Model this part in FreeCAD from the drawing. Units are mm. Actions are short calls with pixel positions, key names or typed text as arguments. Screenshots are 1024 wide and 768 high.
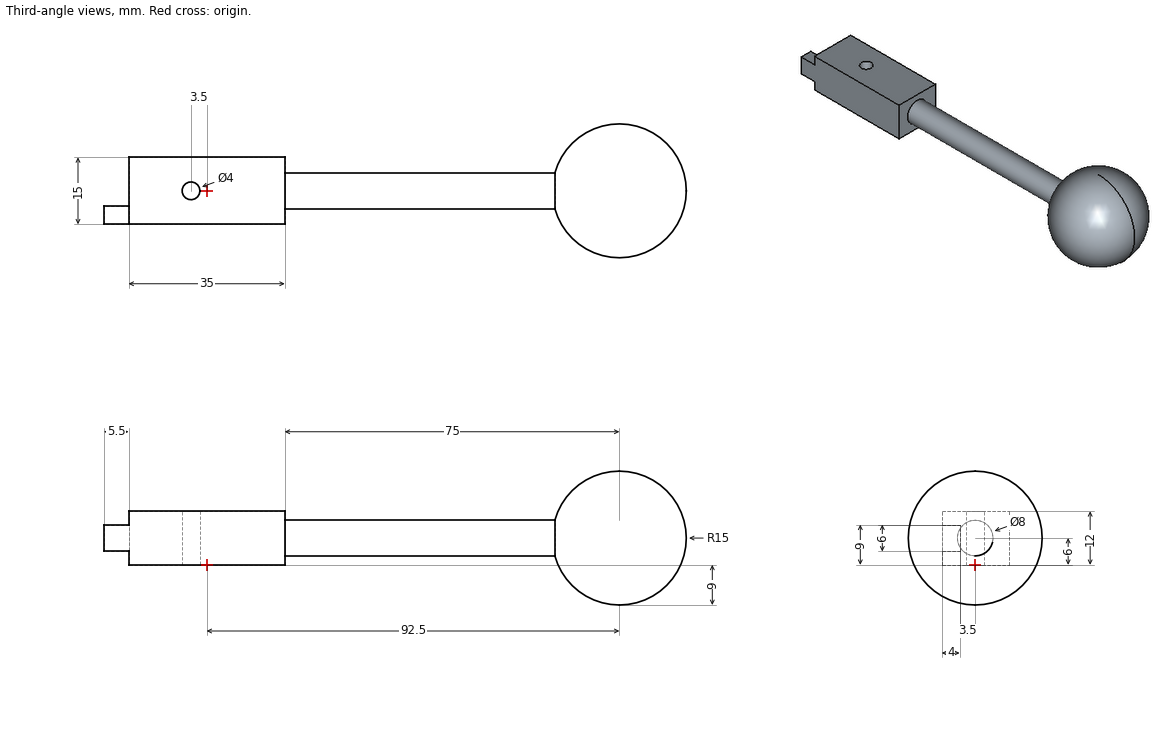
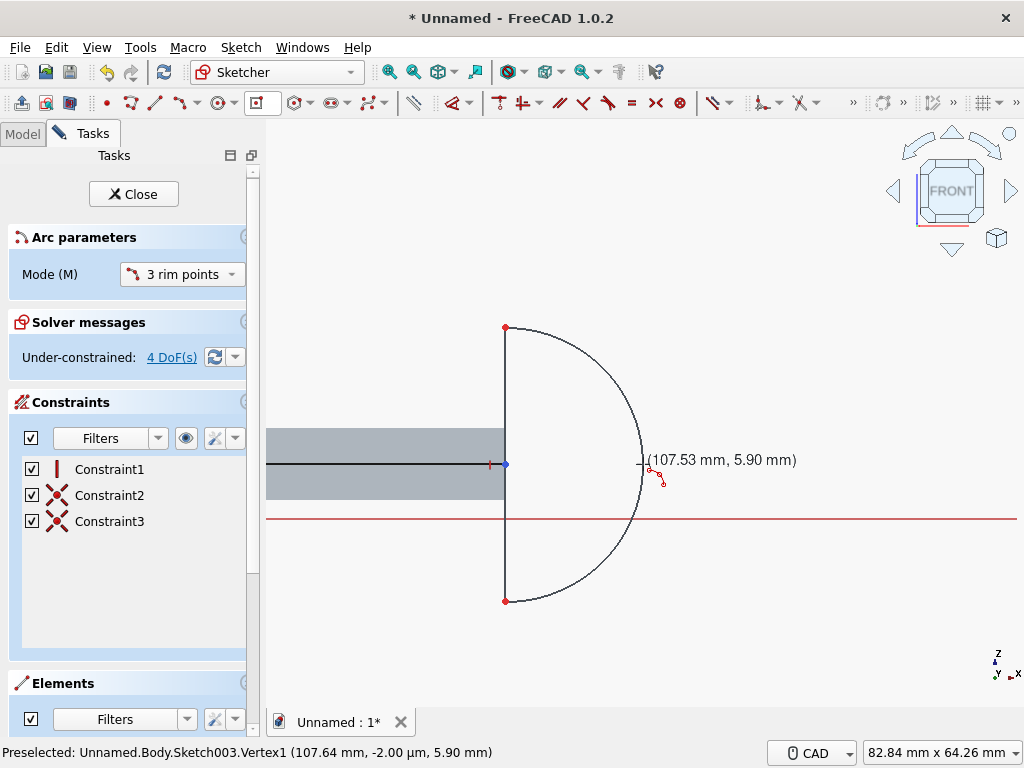
click(156, 104)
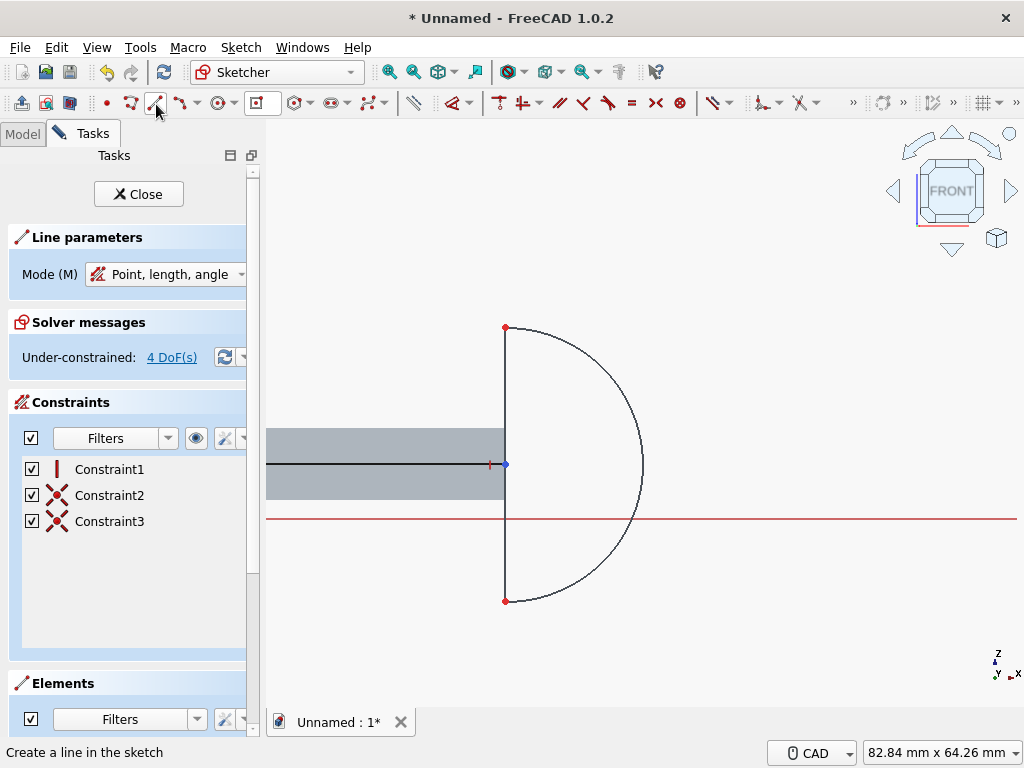
click(505, 299)
click(505, 217)
key(Escape)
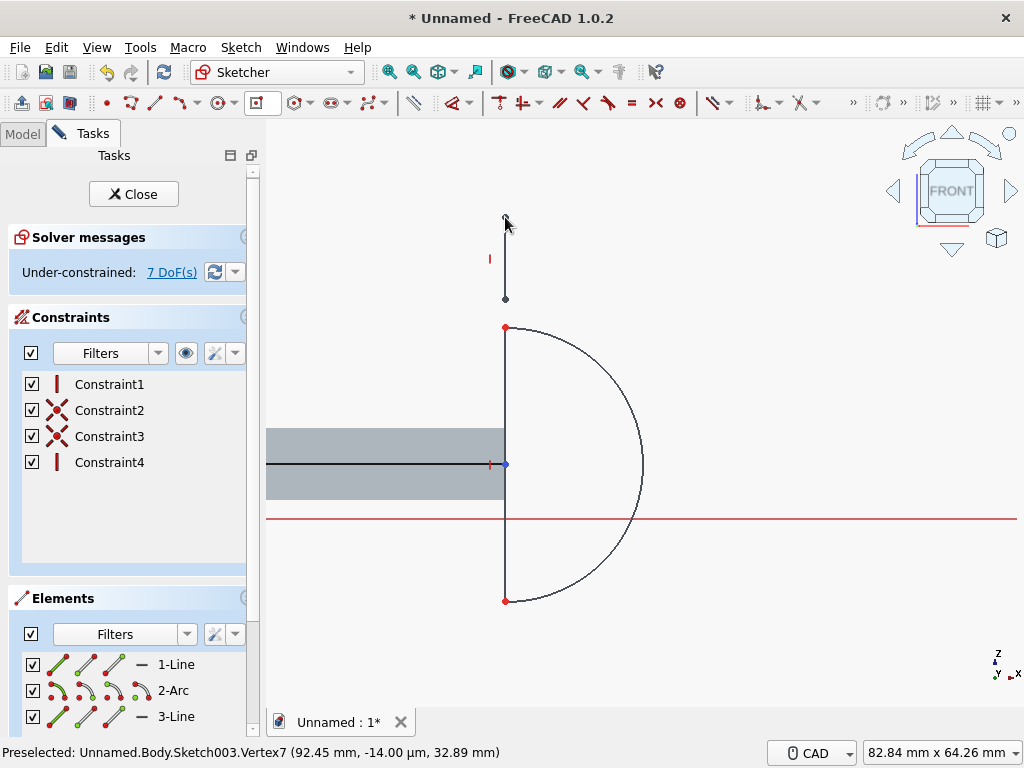
click(505, 275)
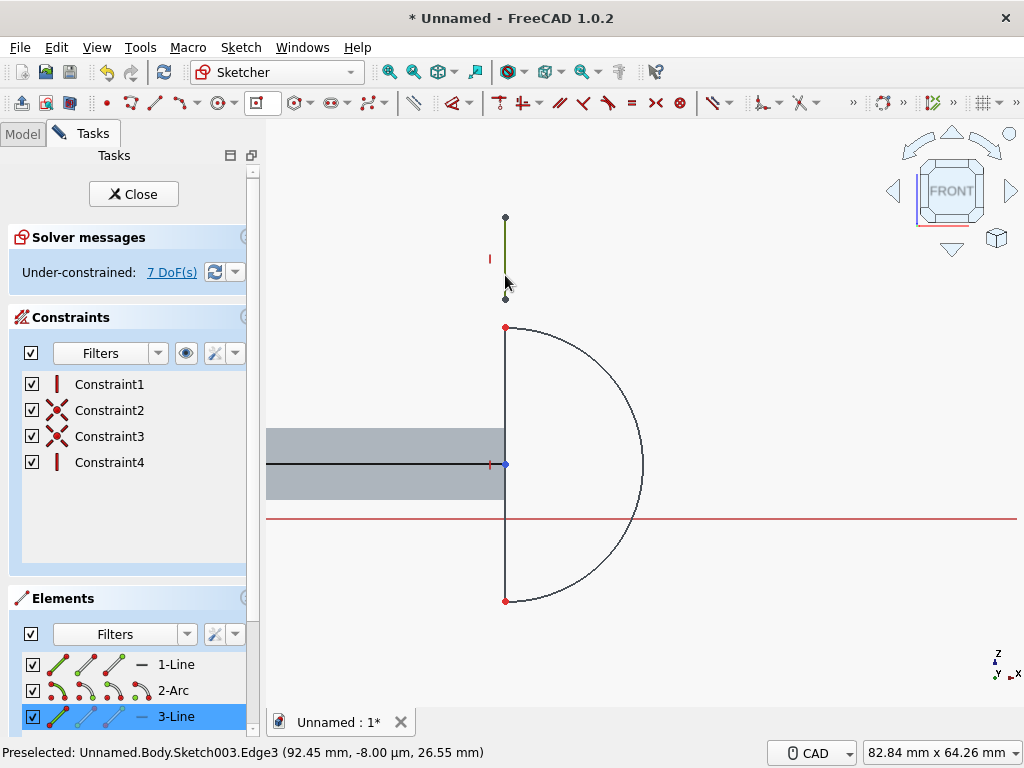
click(414, 104)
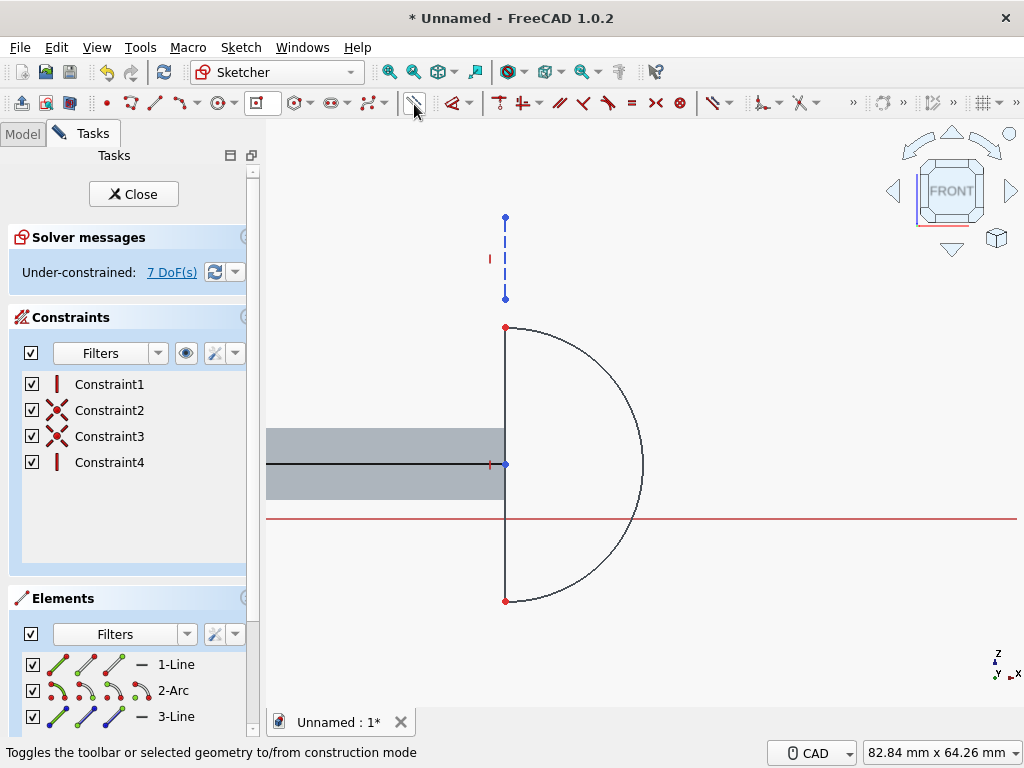
click(452, 104)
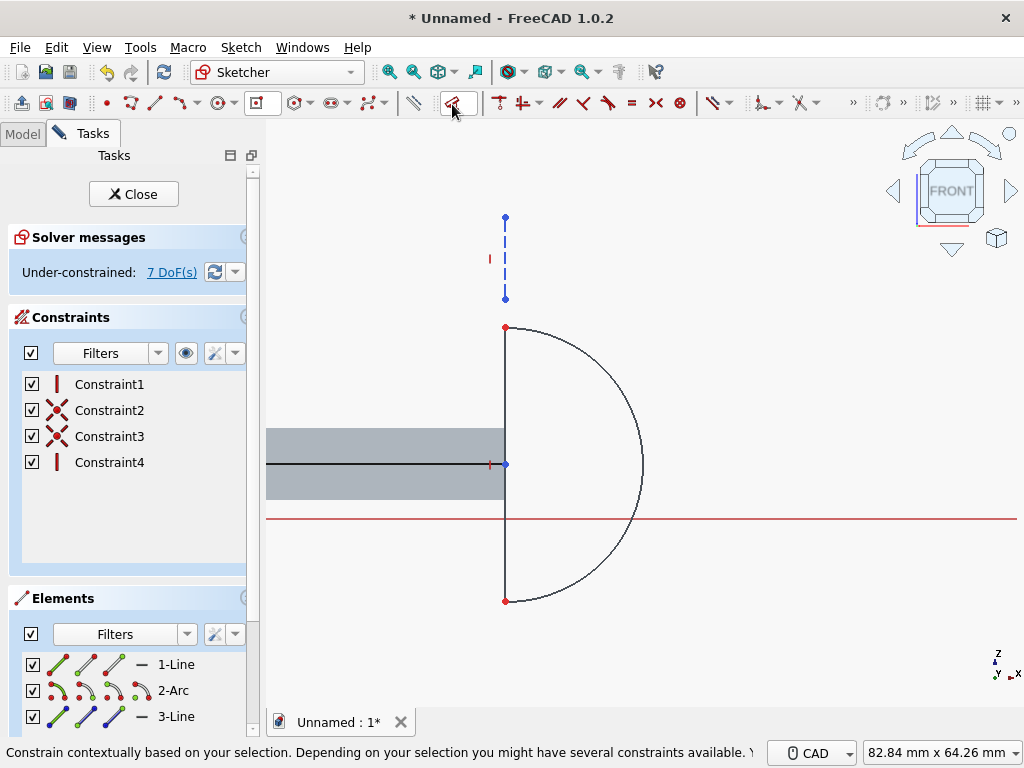
click(617, 546)
click(643, 565)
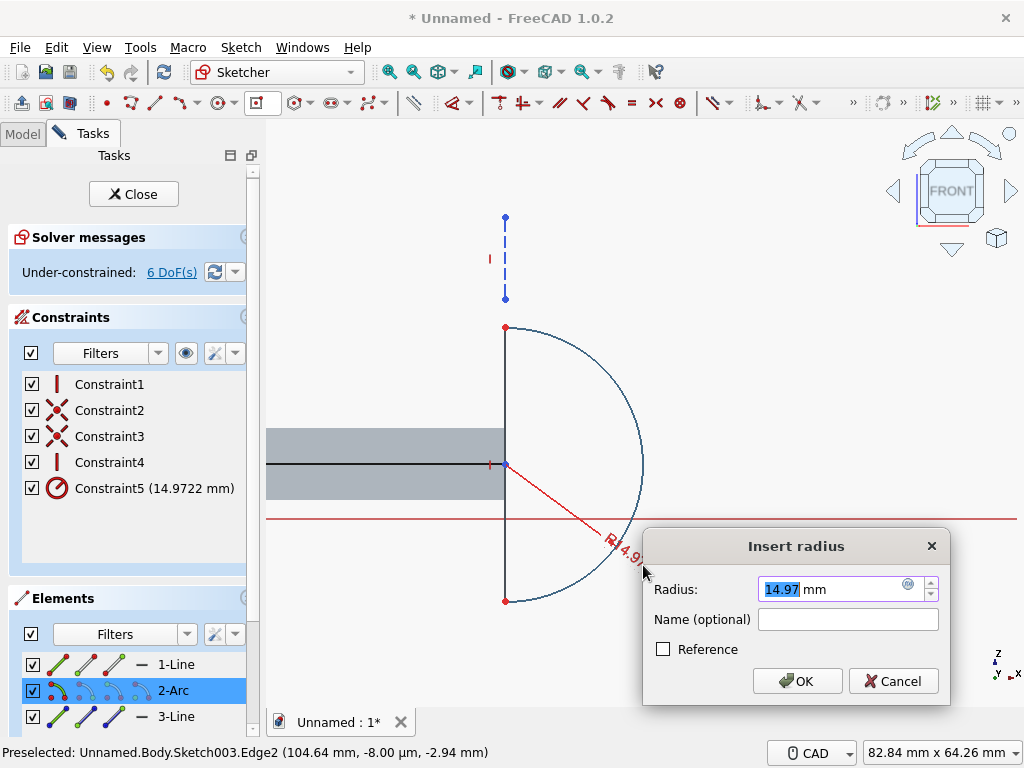
text(15)
key(Return)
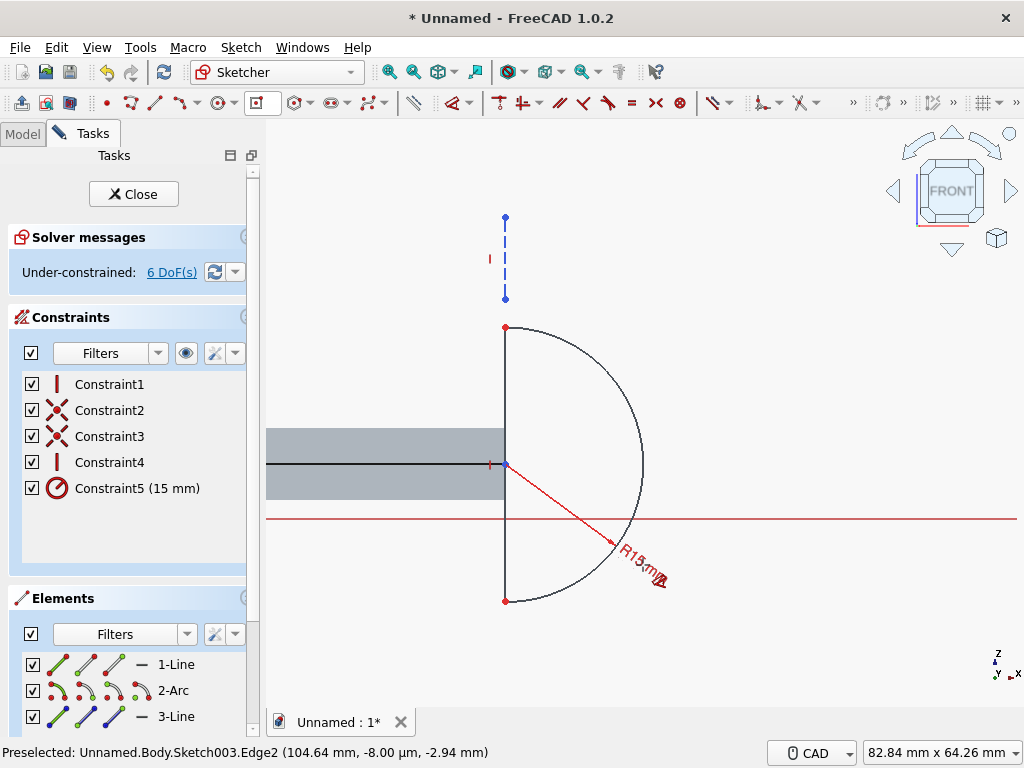
click(505, 602)
click(539, 560)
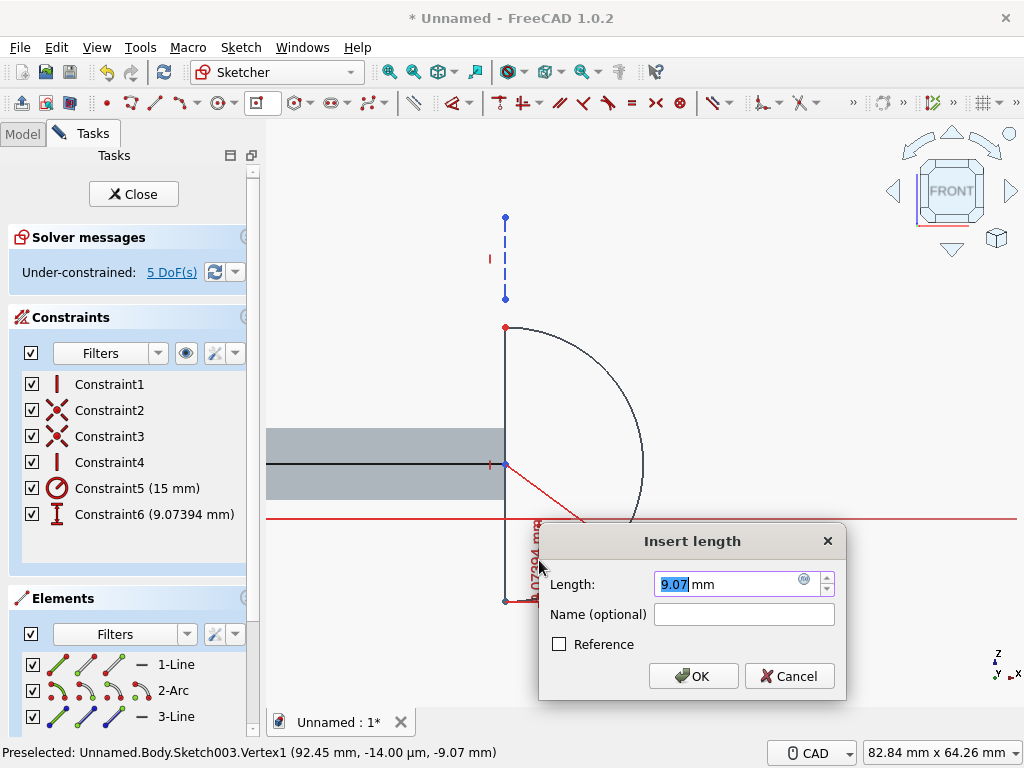
text(9)
key(Return)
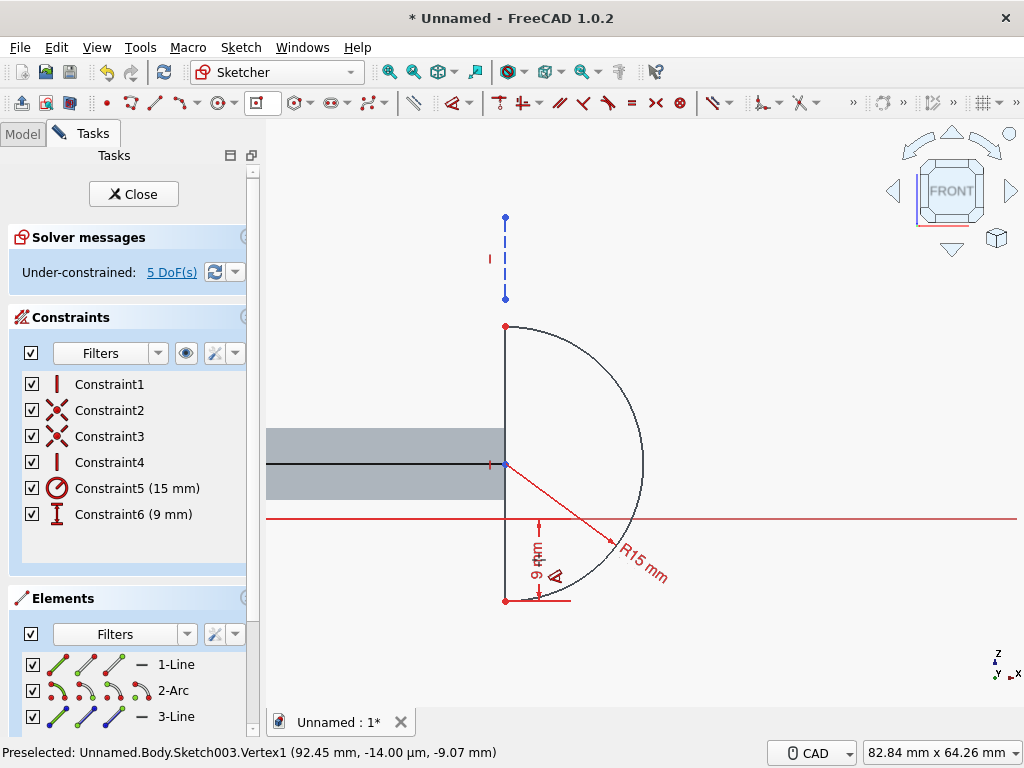
click(505, 601)
click(399, 635)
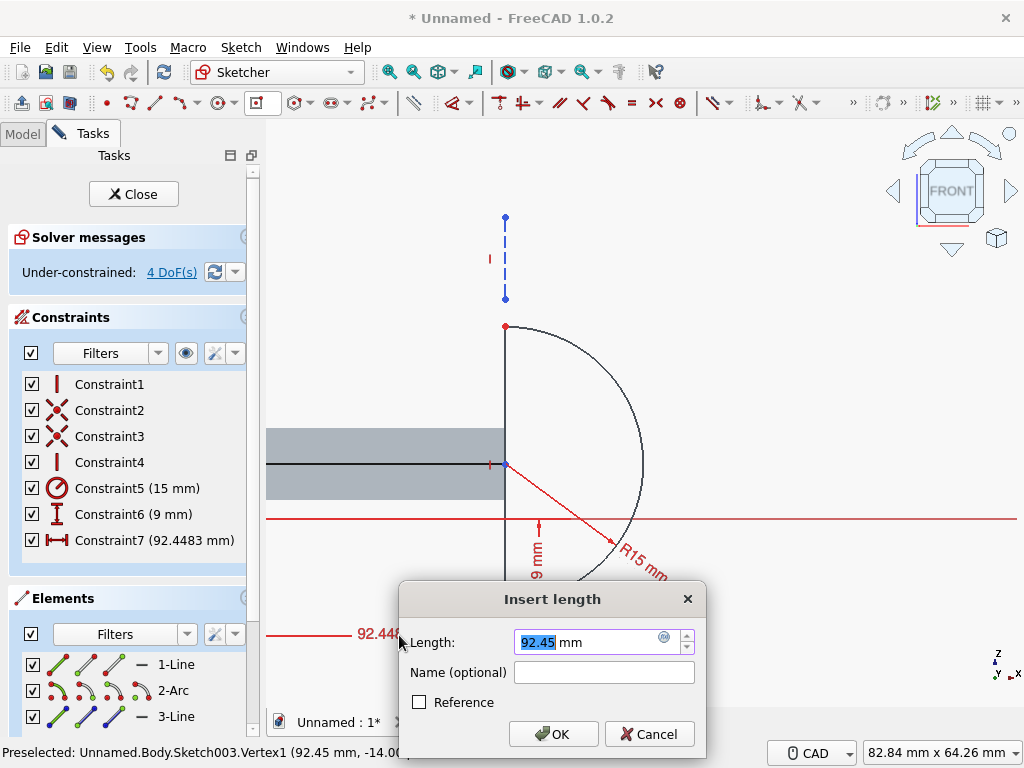
text(92.5)
key(Return)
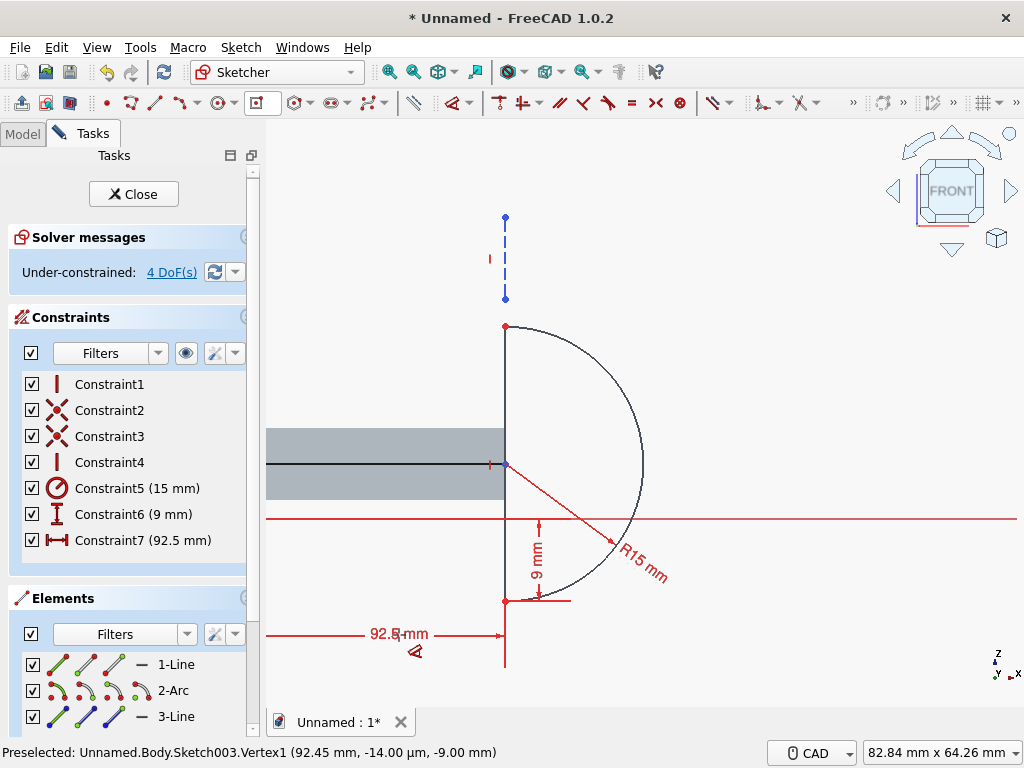
click(505, 300)
click(399, 553)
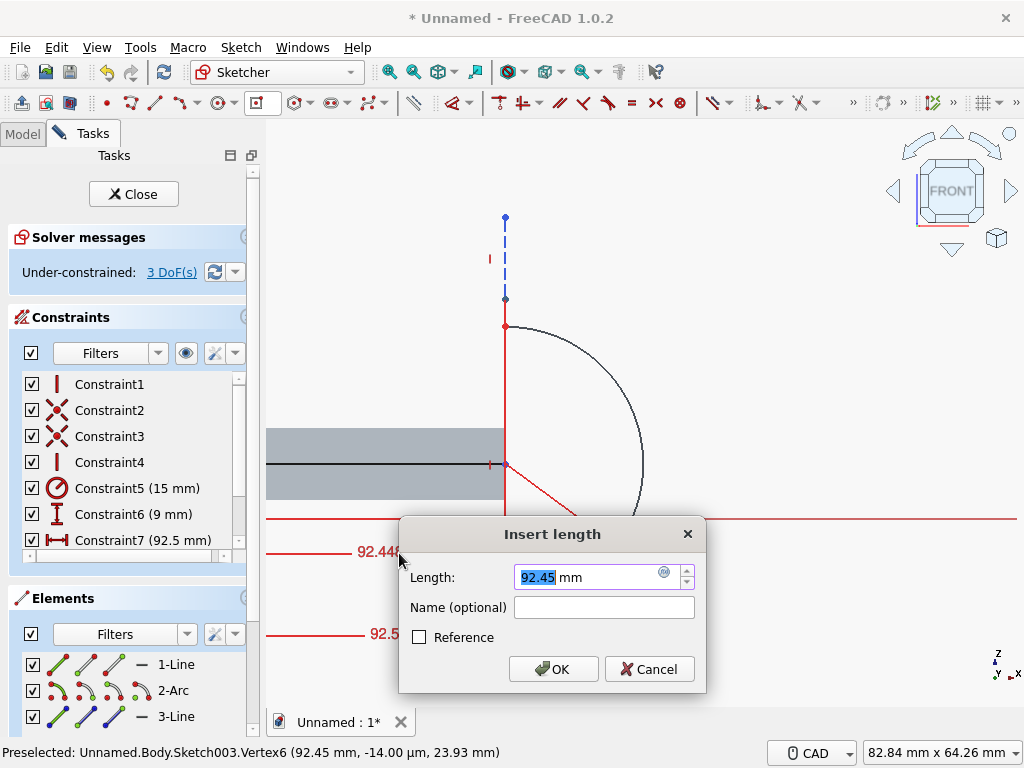
text(92.5)
key(Return)